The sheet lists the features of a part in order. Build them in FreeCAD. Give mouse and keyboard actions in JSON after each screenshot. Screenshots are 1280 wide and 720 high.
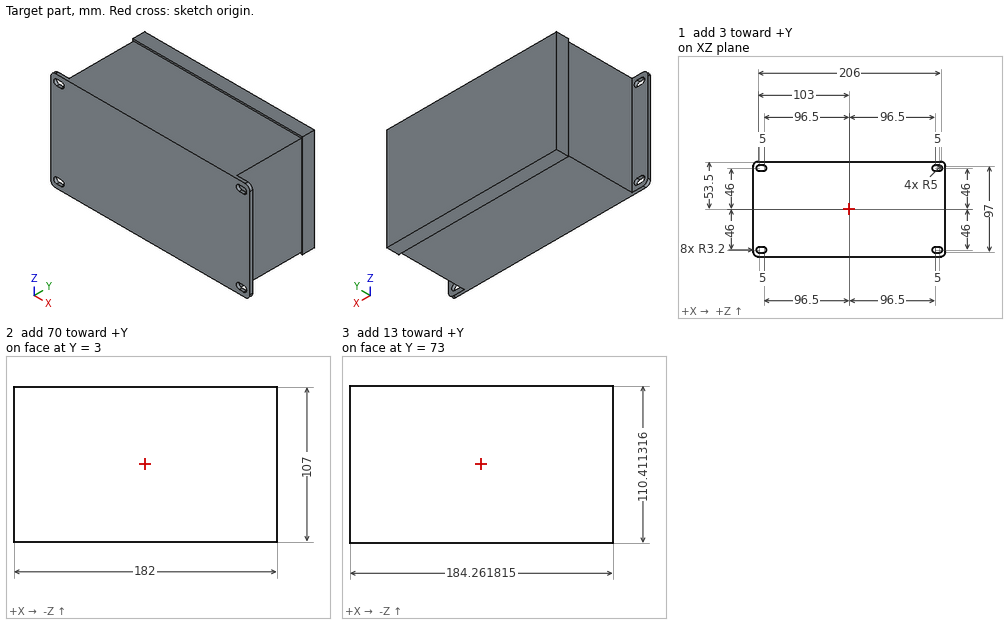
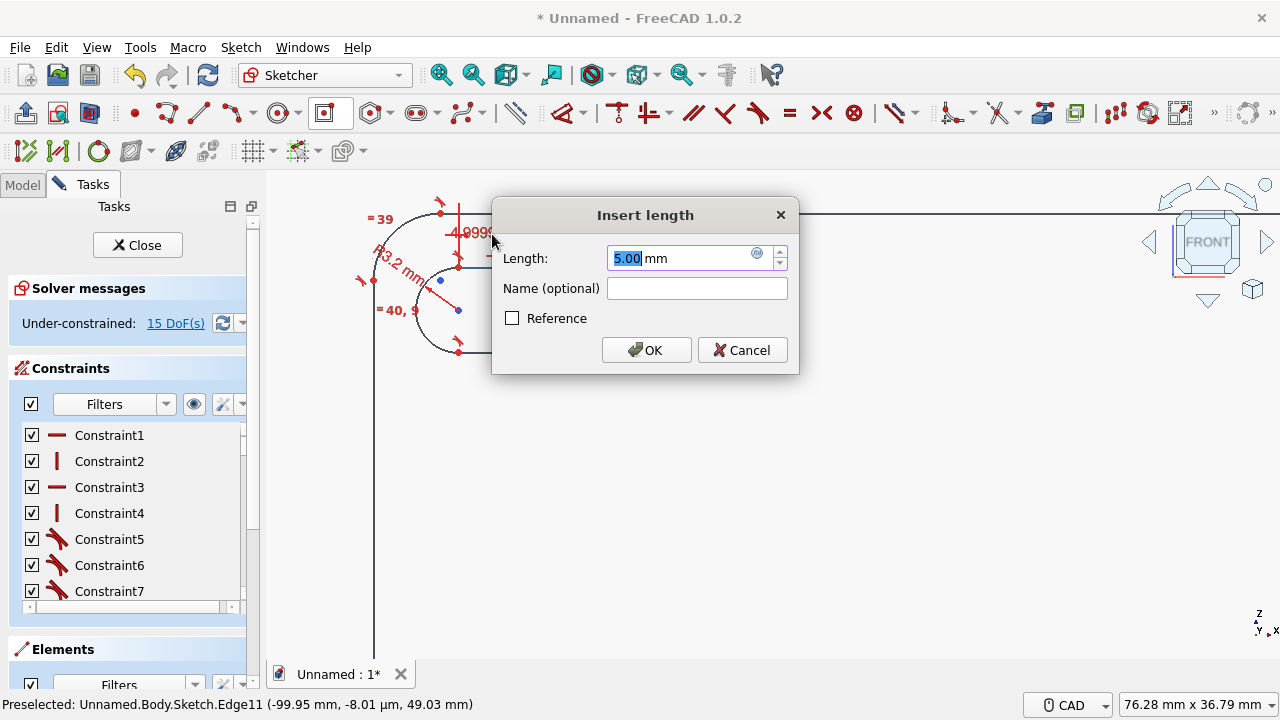
{"action": "type", "text": "5"}
{"action": "key", "text": "Return"}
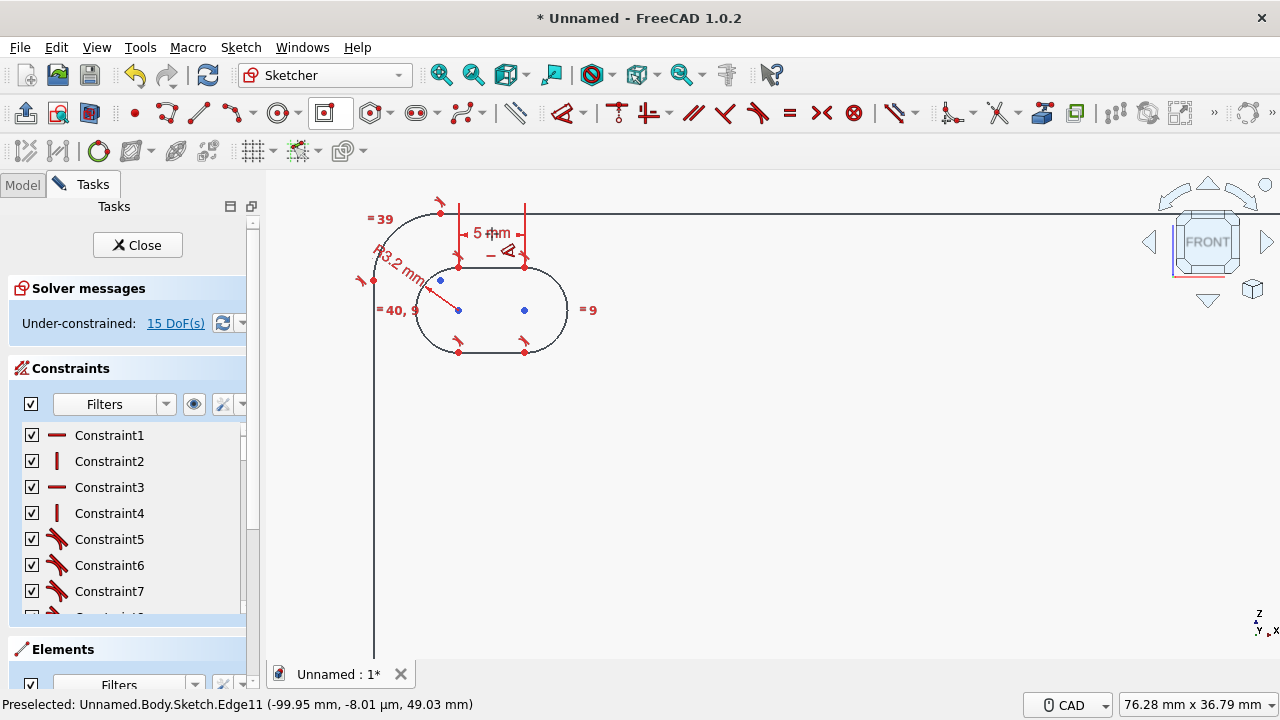
{"action": "scroll", "coordinate": [426, 287], "scroll_direction": "down", "scroll_amount": 8}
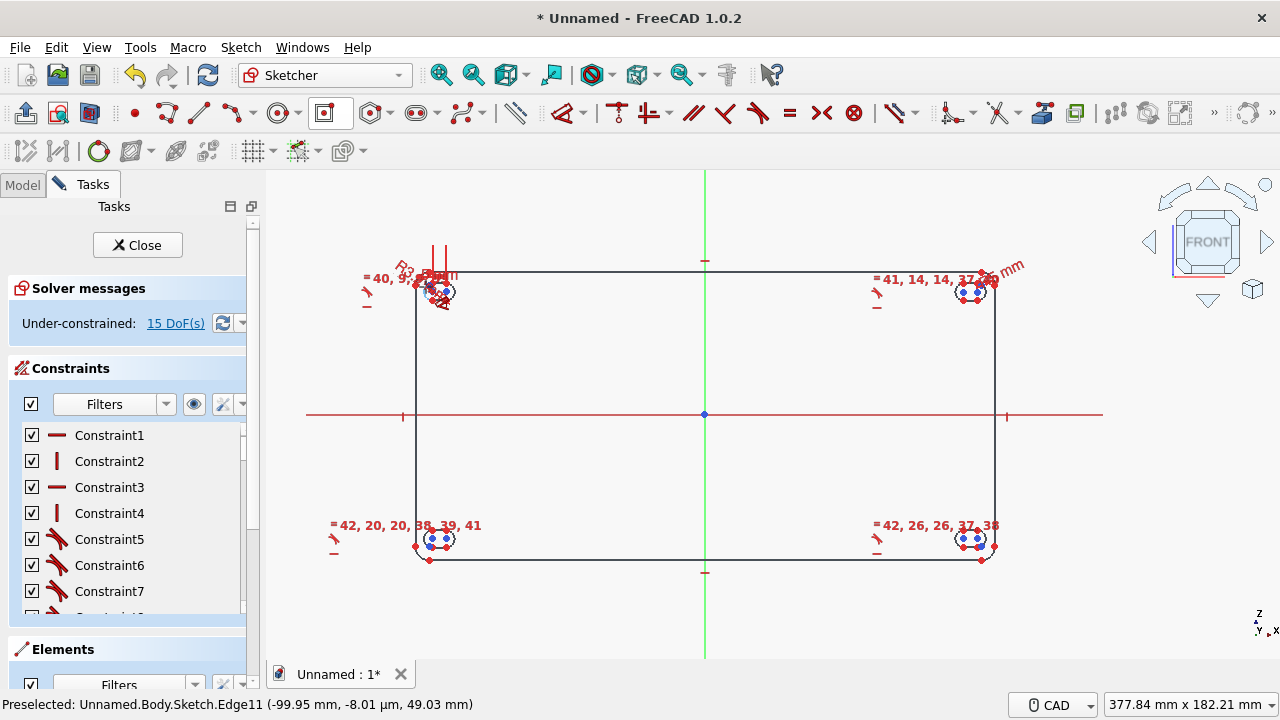
{"action": "scroll", "coordinate": [968, 283], "scroll_direction": "up", "scroll_amount": 7}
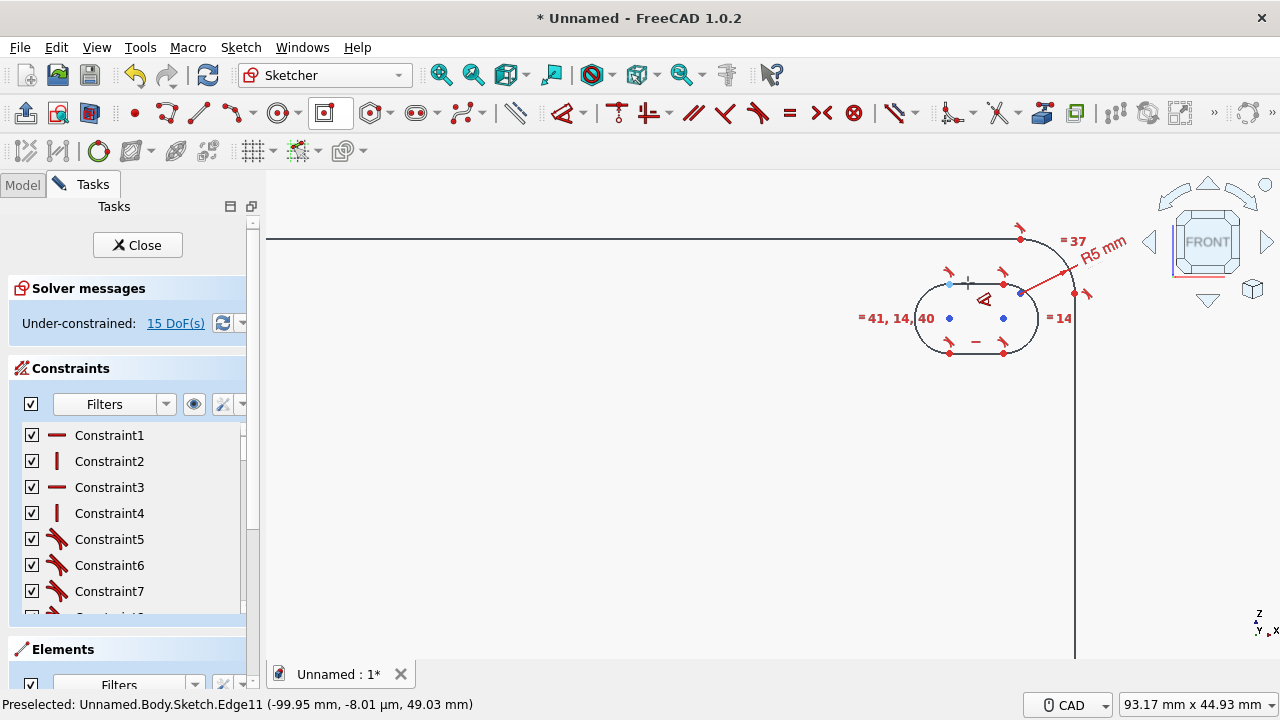
{"action": "left_click", "coordinate": [966, 284]}
{"action": "left_click", "coordinate": [976, 318]}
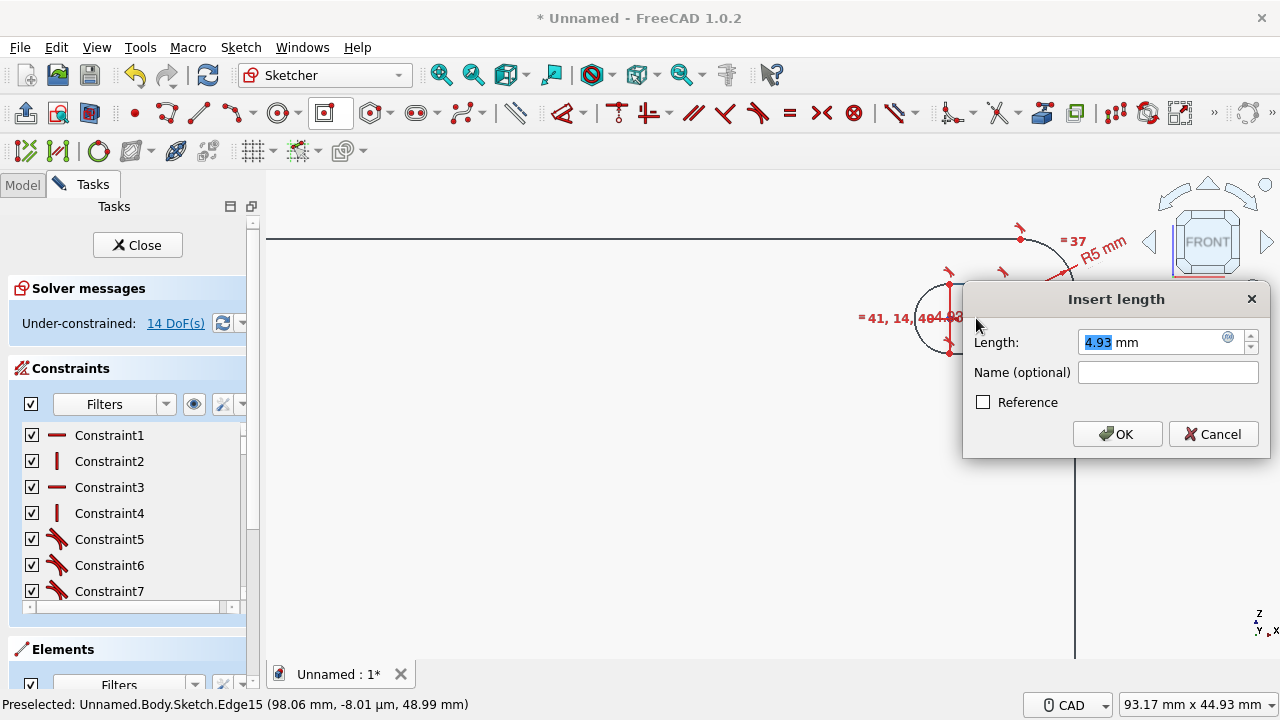
{"action": "type", "text": "5"}
{"action": "key", "text": "Return"}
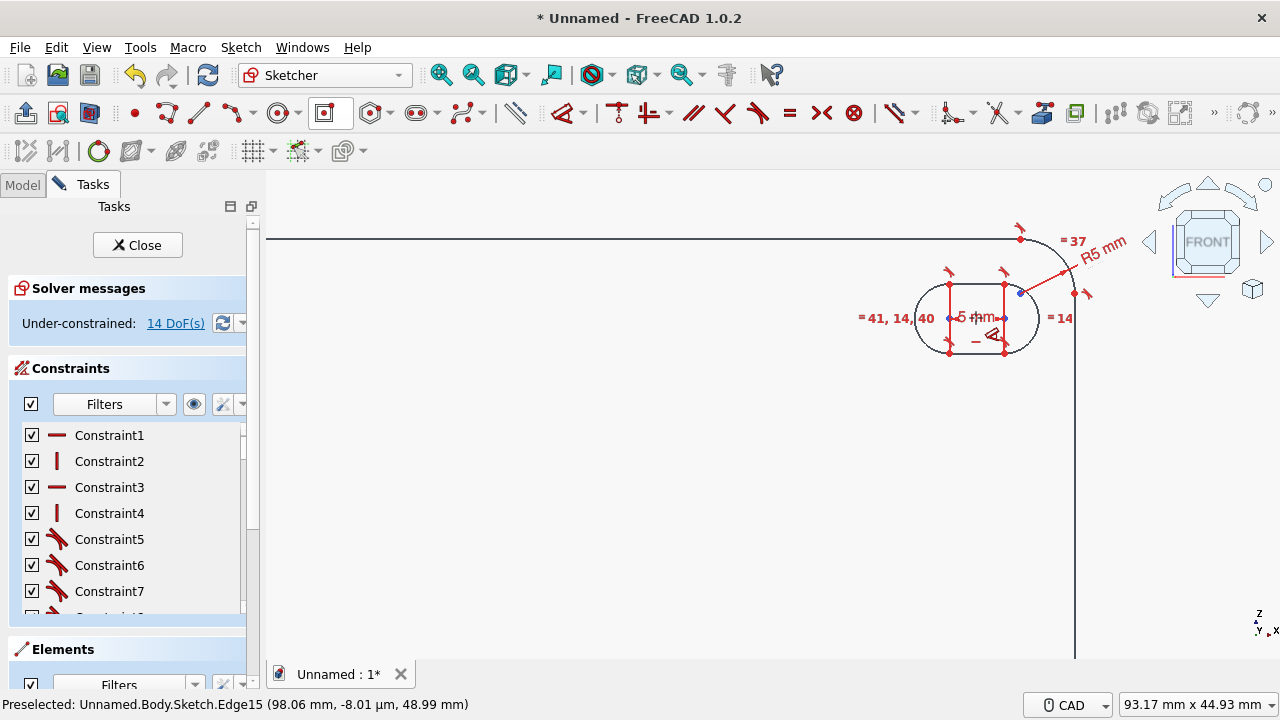
{"action": "scroll", "coordinate": [968, 283], "scroll_direction": "down", "scroll_amount": 7}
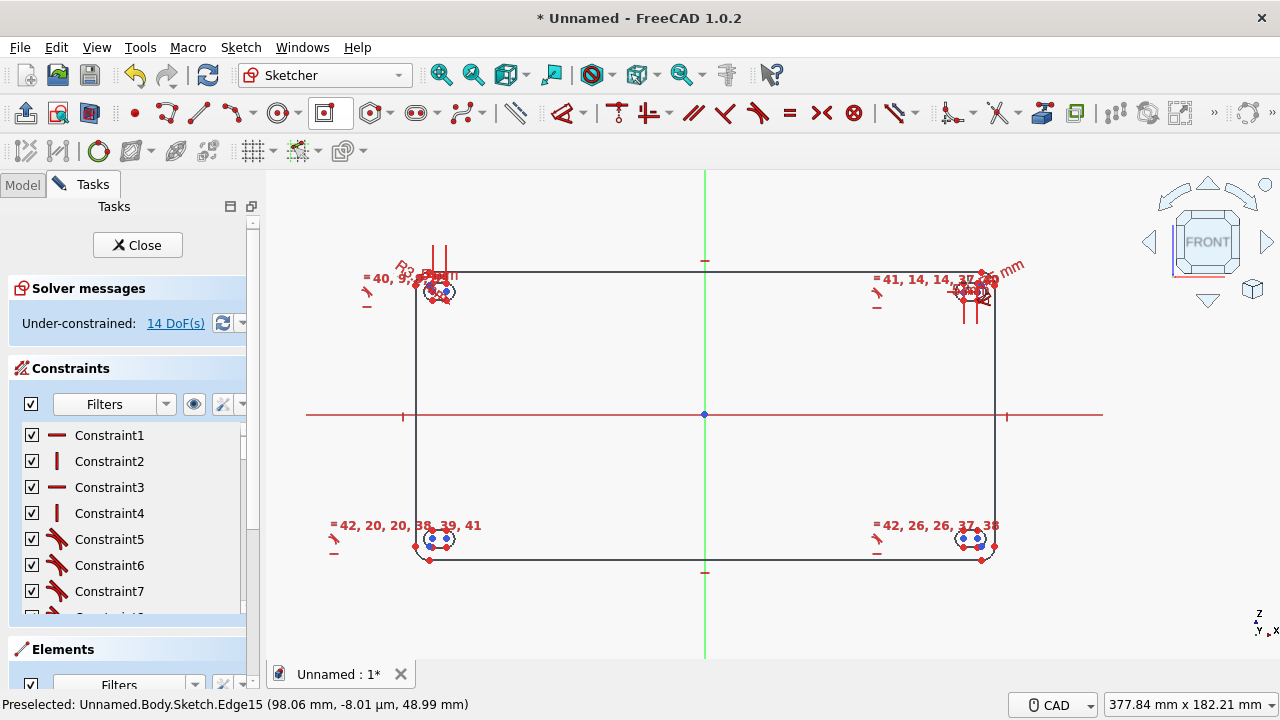
{"action": "scroll", "coordinate": [436, 530], "scroll_direction": "up", "scroll_amount": 7}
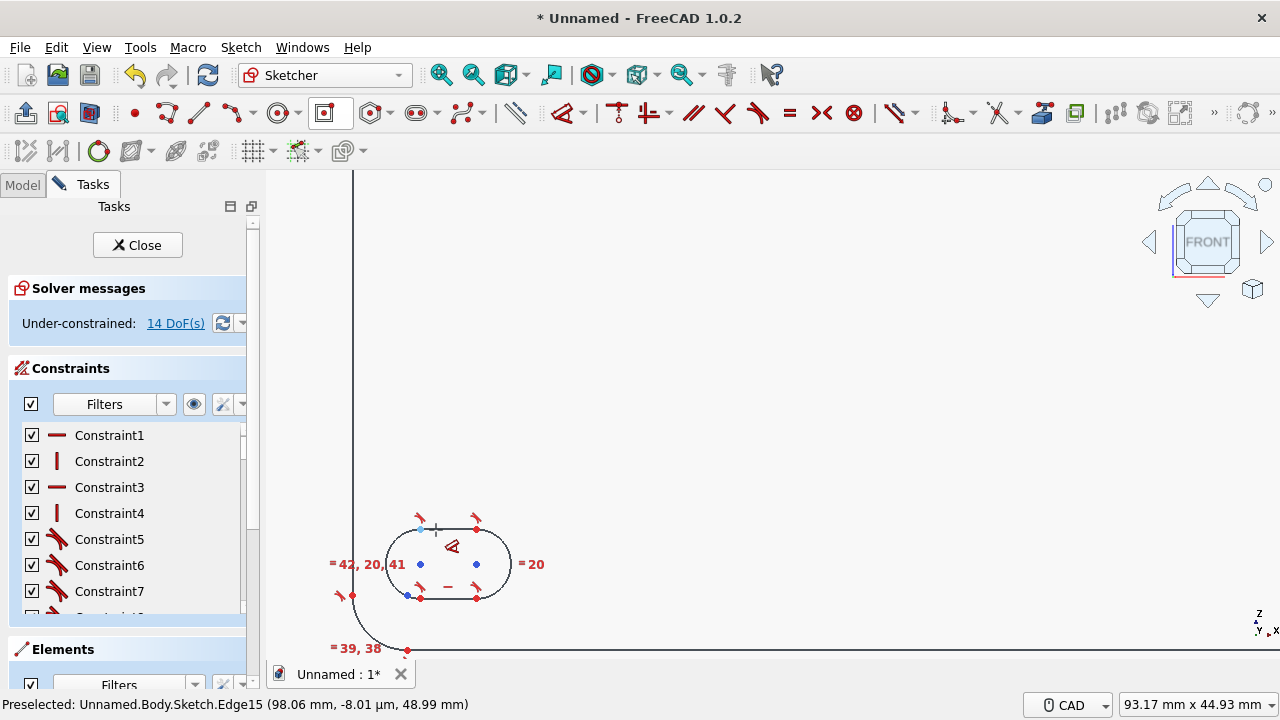
{"action": "left_click", "coordinate": [437, 529]}
{"action": "left_click", "coordinate": [448, 563]}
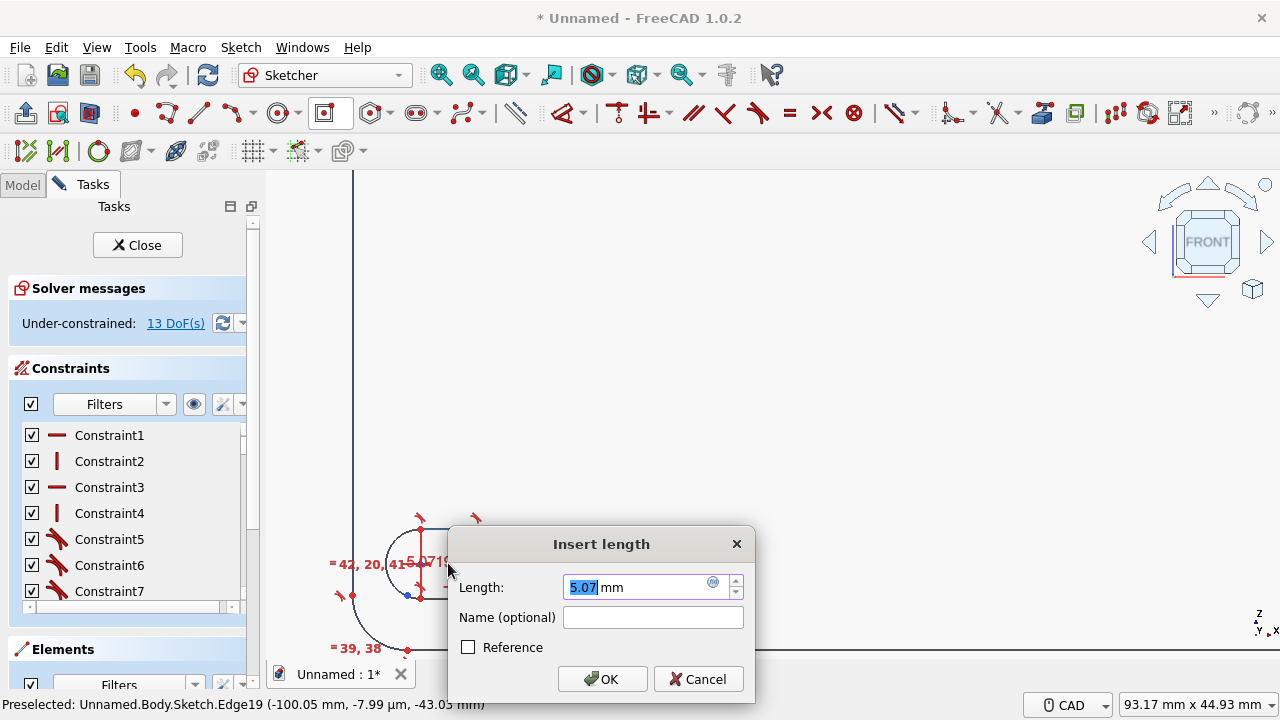
{"action": "type", "text": "5"}
{"action": "key", "text": "Return"}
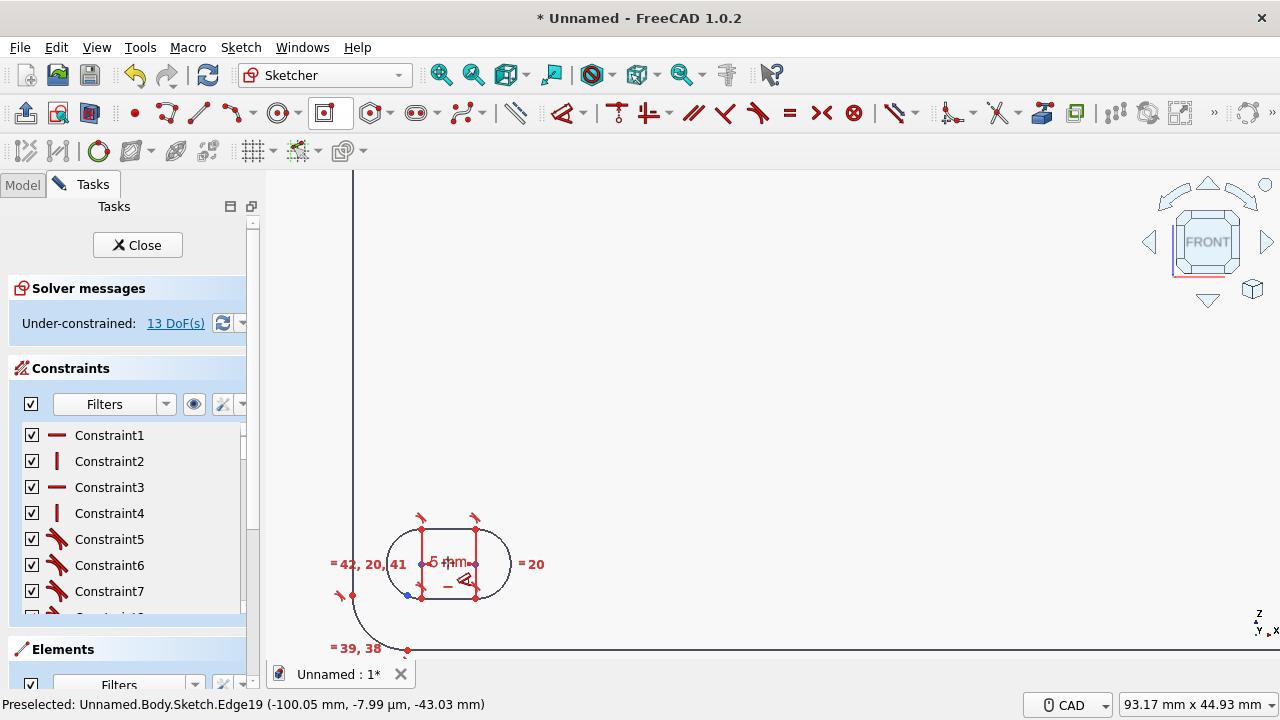
{"action": "scroll", "coordinate": [436, 530], "scroll_direction": "down", "scroll_amount": 7}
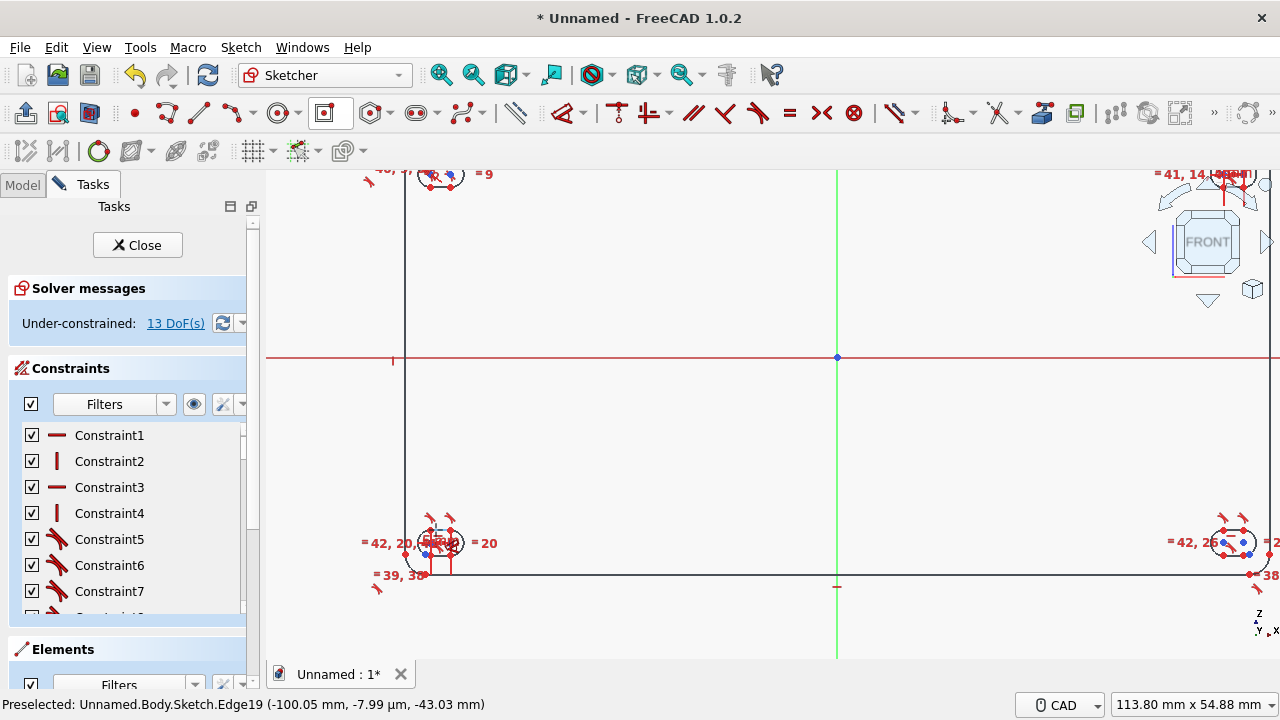
{"action": "scroll", "coordinate": [968, 530], "scroll_direction": "up", "scroll_amount": 7}